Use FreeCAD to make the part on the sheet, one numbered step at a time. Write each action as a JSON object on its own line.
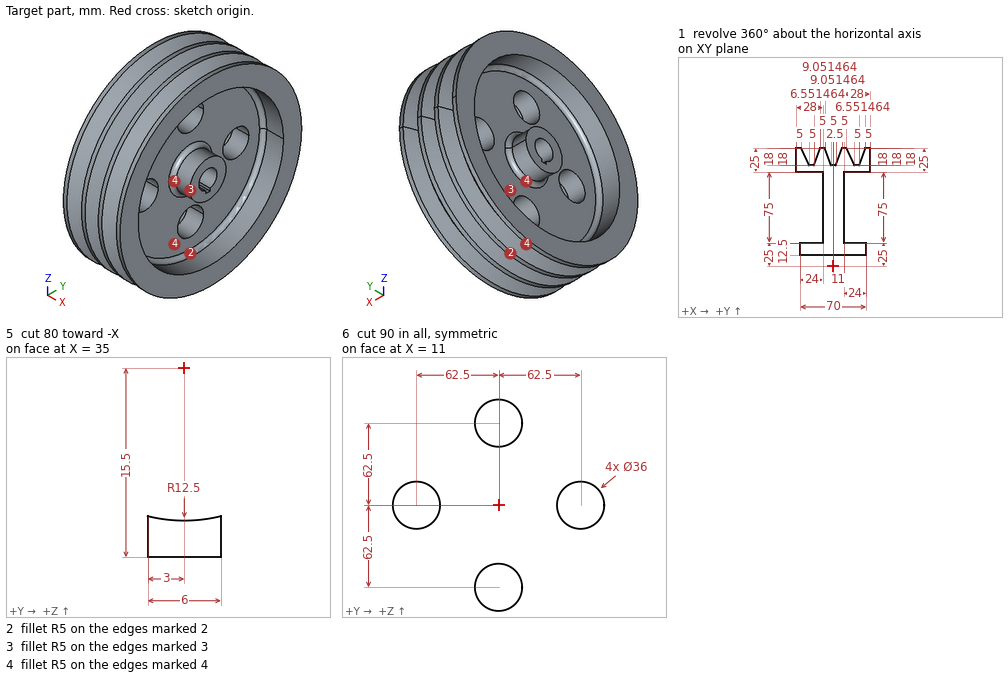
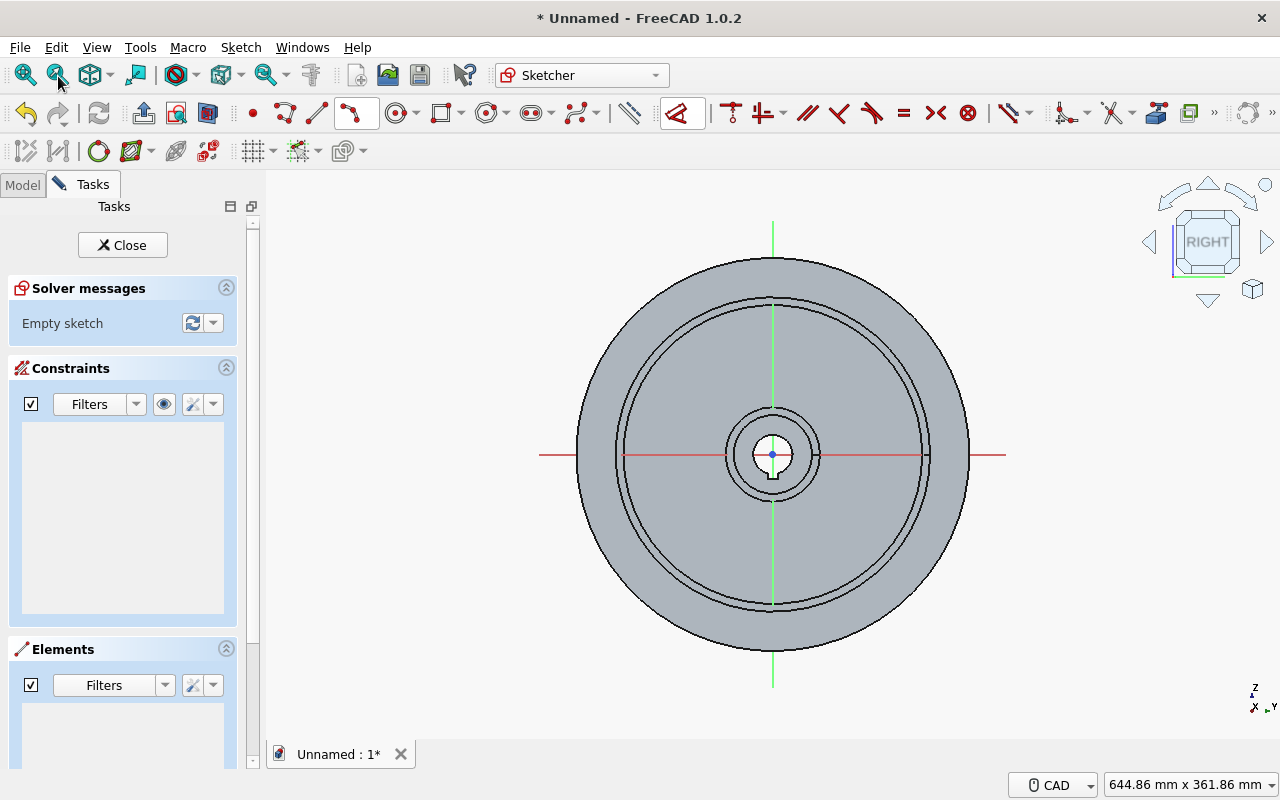
{"action": "scroll", "coordinate": [912, 454], "scroll_direction": "up", "scroll_amount": 2}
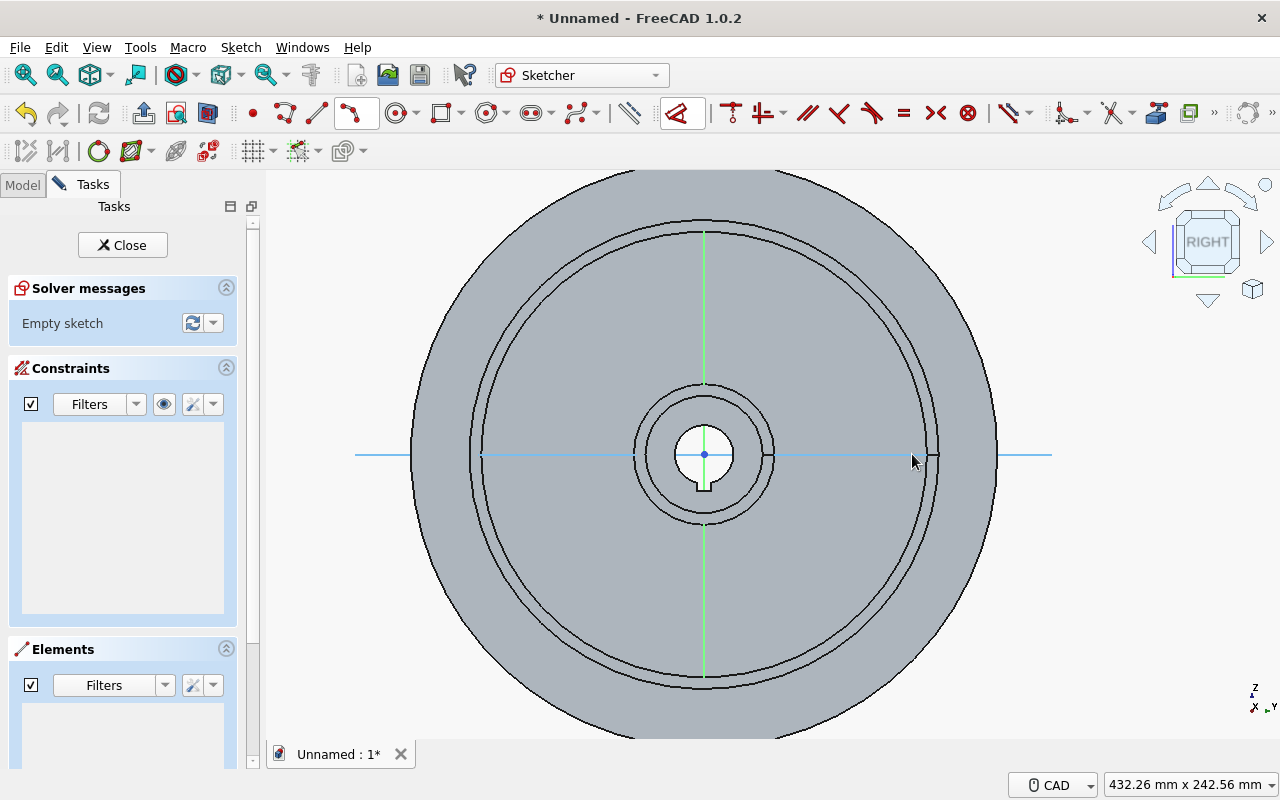
{"action": "left_click", "coordinate": [396, 114]}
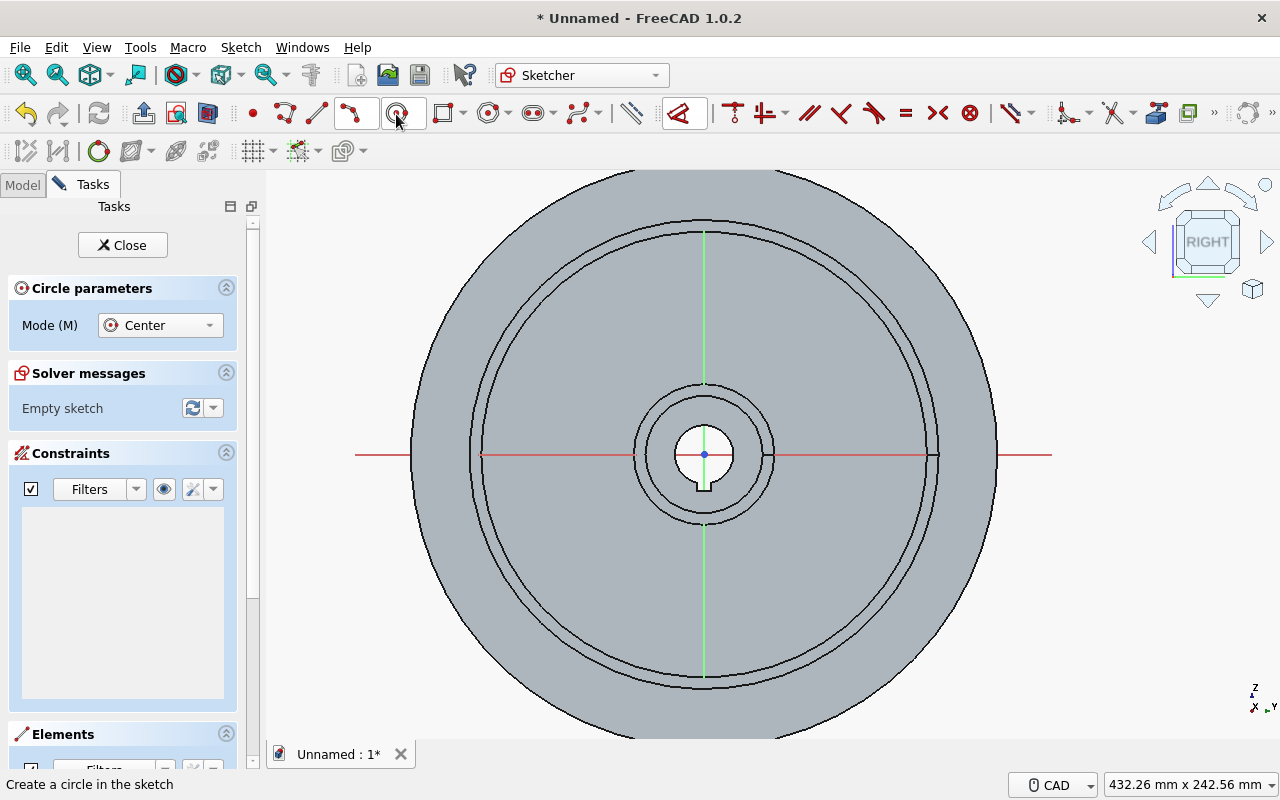
{"action": "left_click", "coordinate": [851, 454]}
{"action": "mouse_move", "coordinate": [881, 425]}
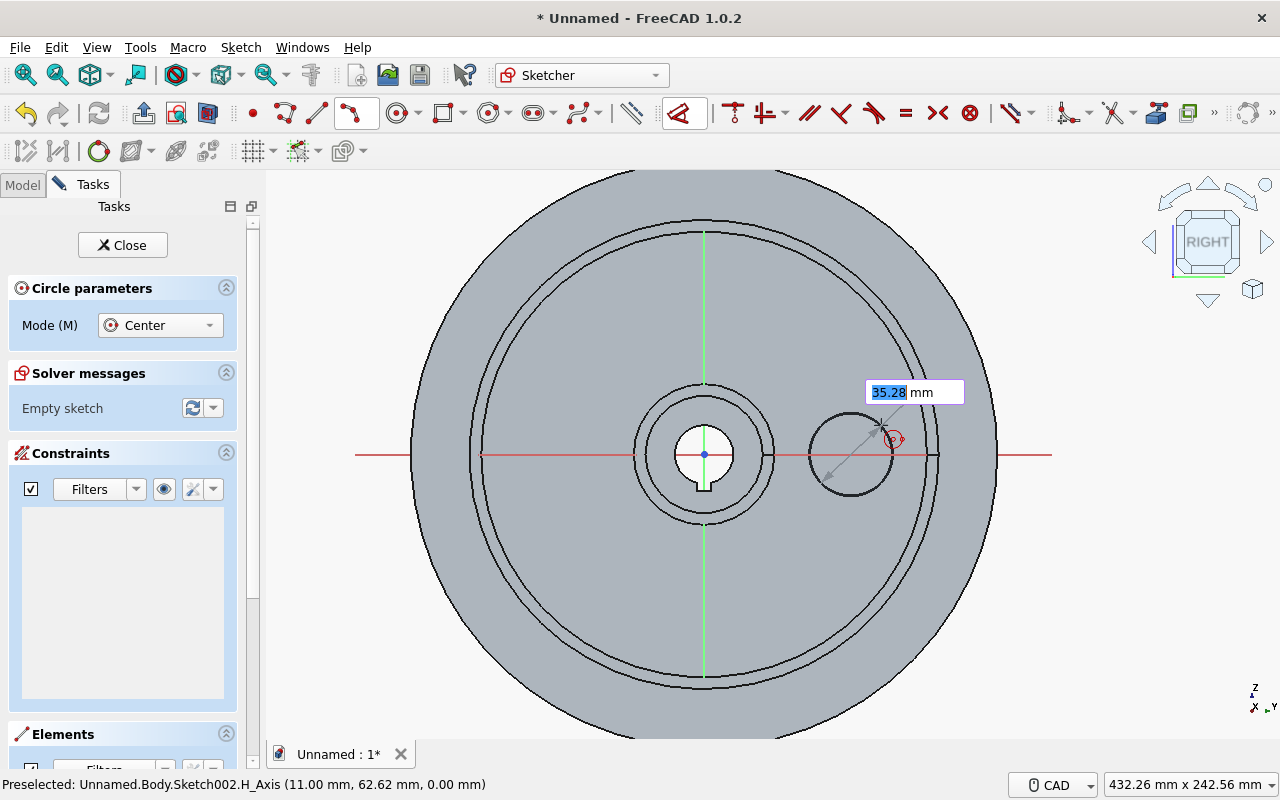
{"action": "type", "text": "36"}
{"action": "key", "text": "Return"}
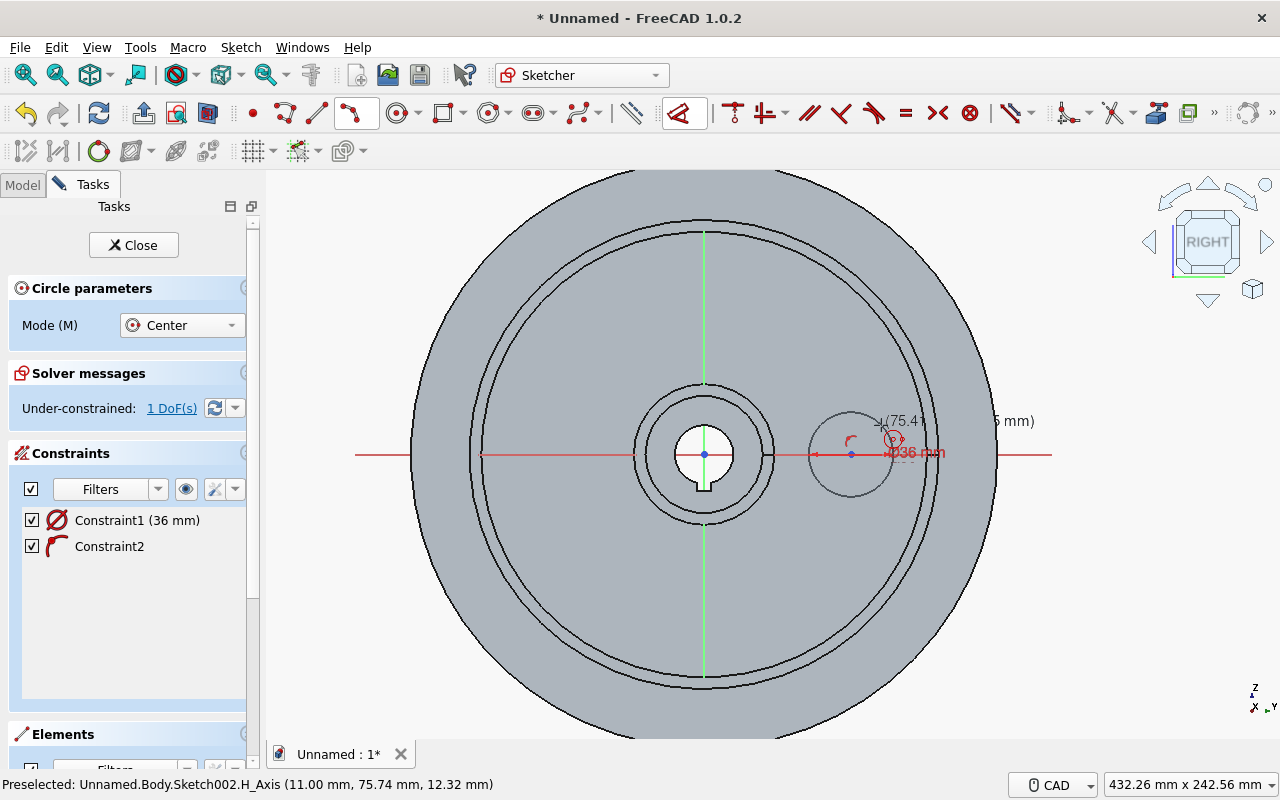
{"action": "left_click", "coordinate": [704, 601]}
{"action": "mouse_move", "coordinate": [734, 571]}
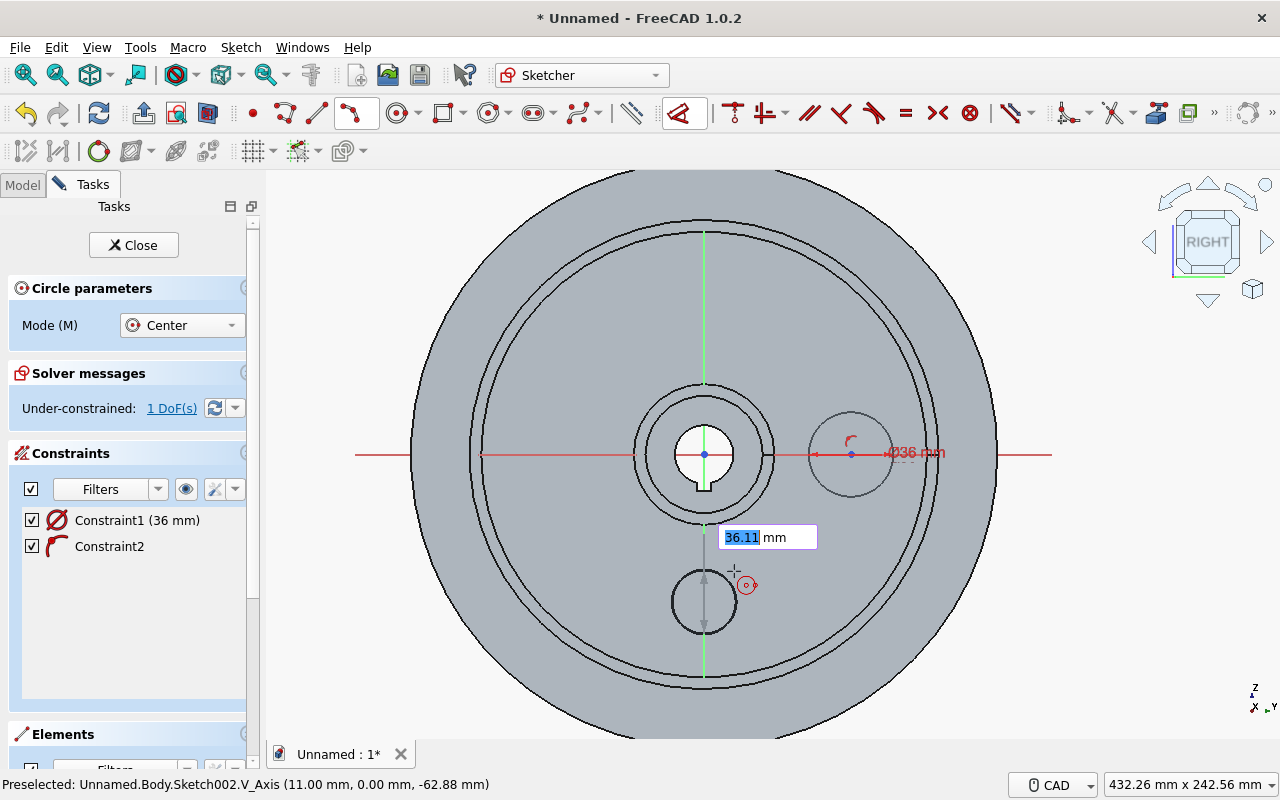
{"action": "type", "text": "36"}
{"action": "key", "text": "Return"}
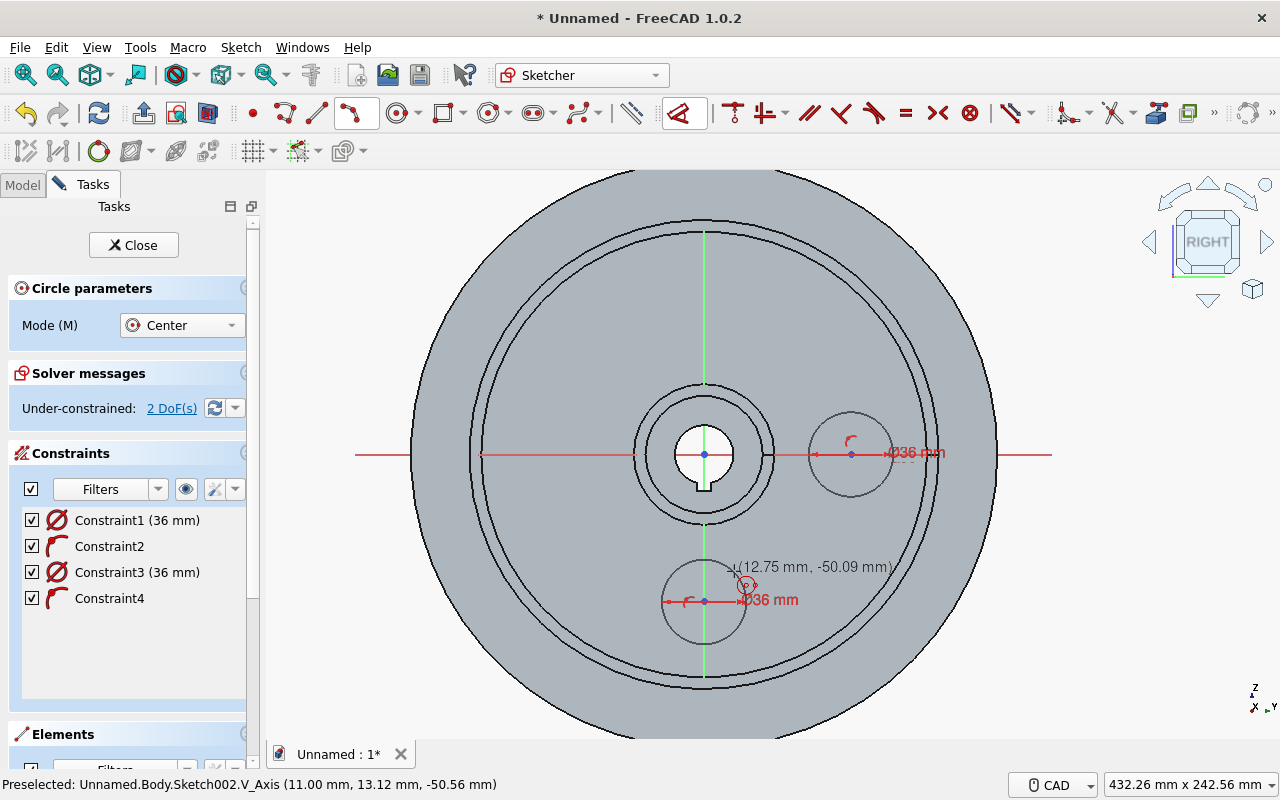
{"action": "left_click", "coordinate": [557, 454]}
{"action": "mouse_move", "coordinate": [587, 425]}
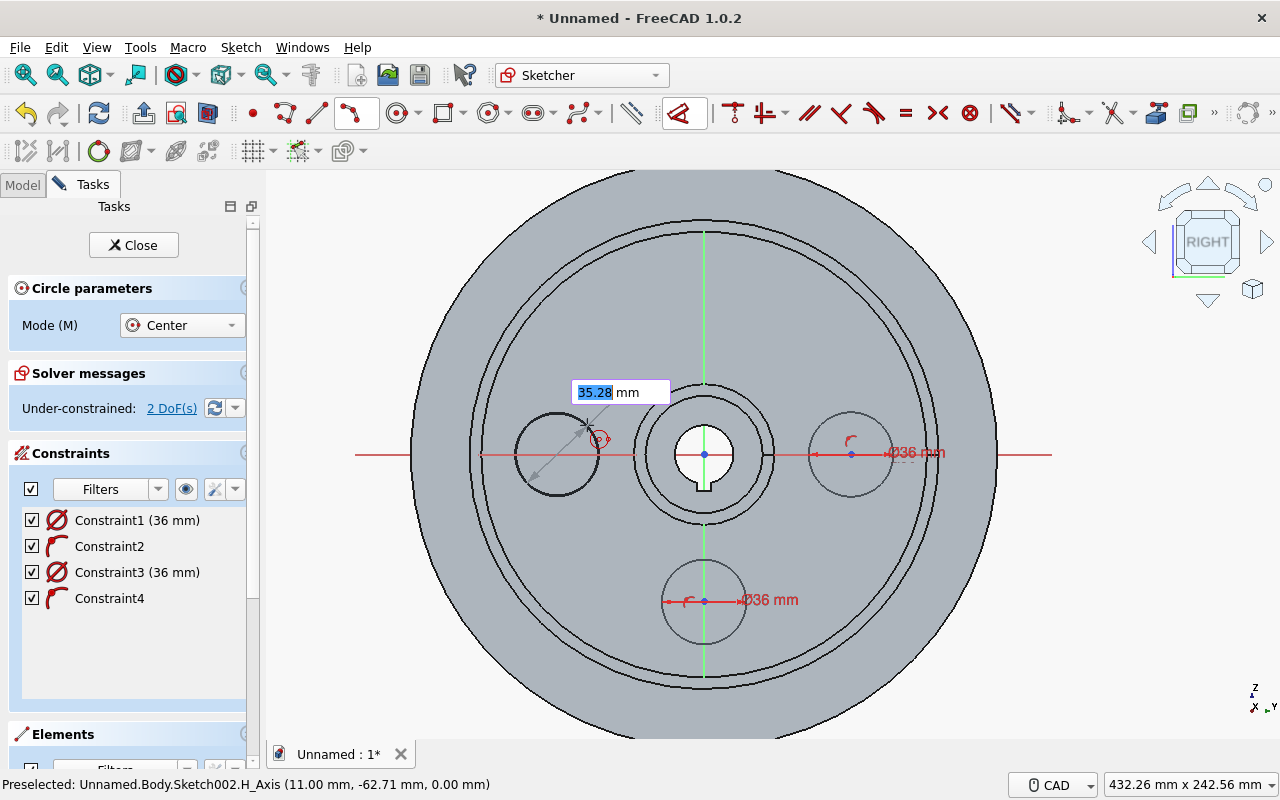
{"action": "type", "text": "36"}
{"action": "key", "text": "Return"}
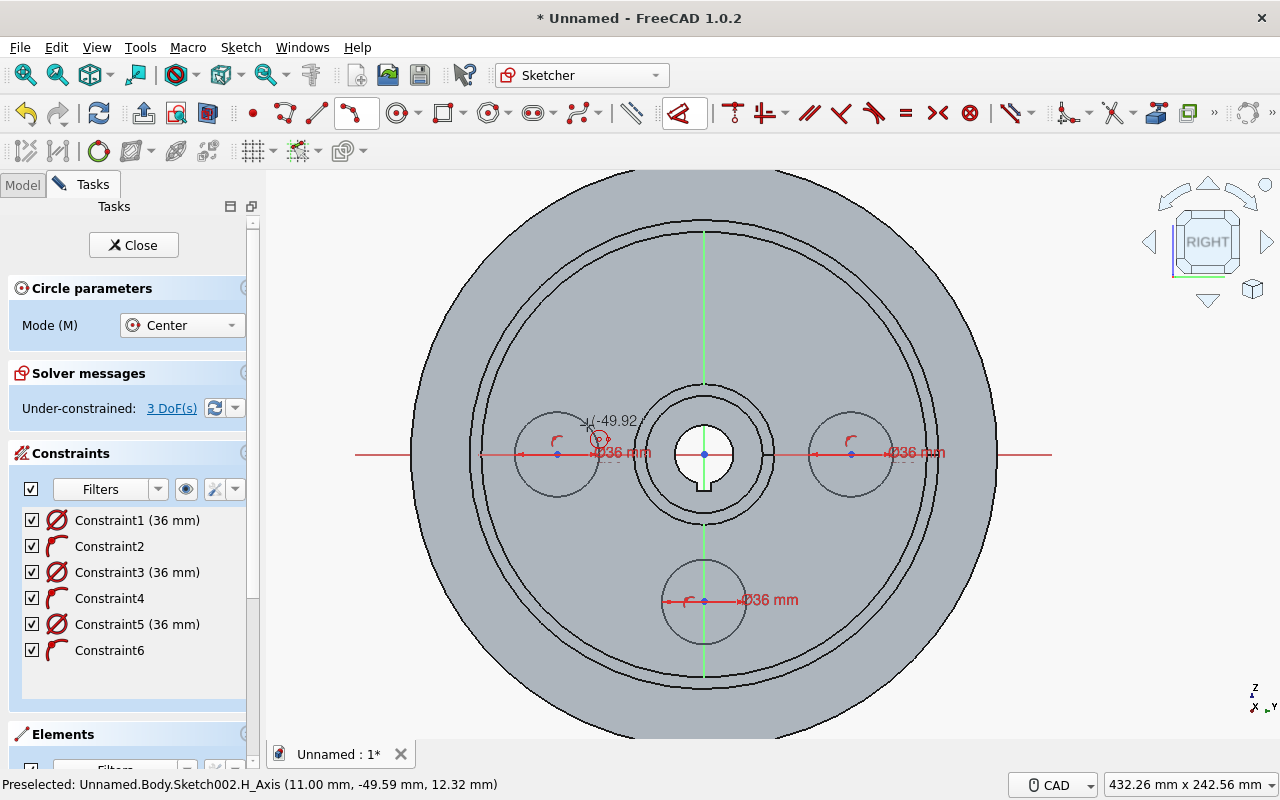
{"action": "left_click", "coordinate": [704, 308]}
{"action": "mouse_move", "coordinate": [734, 278]}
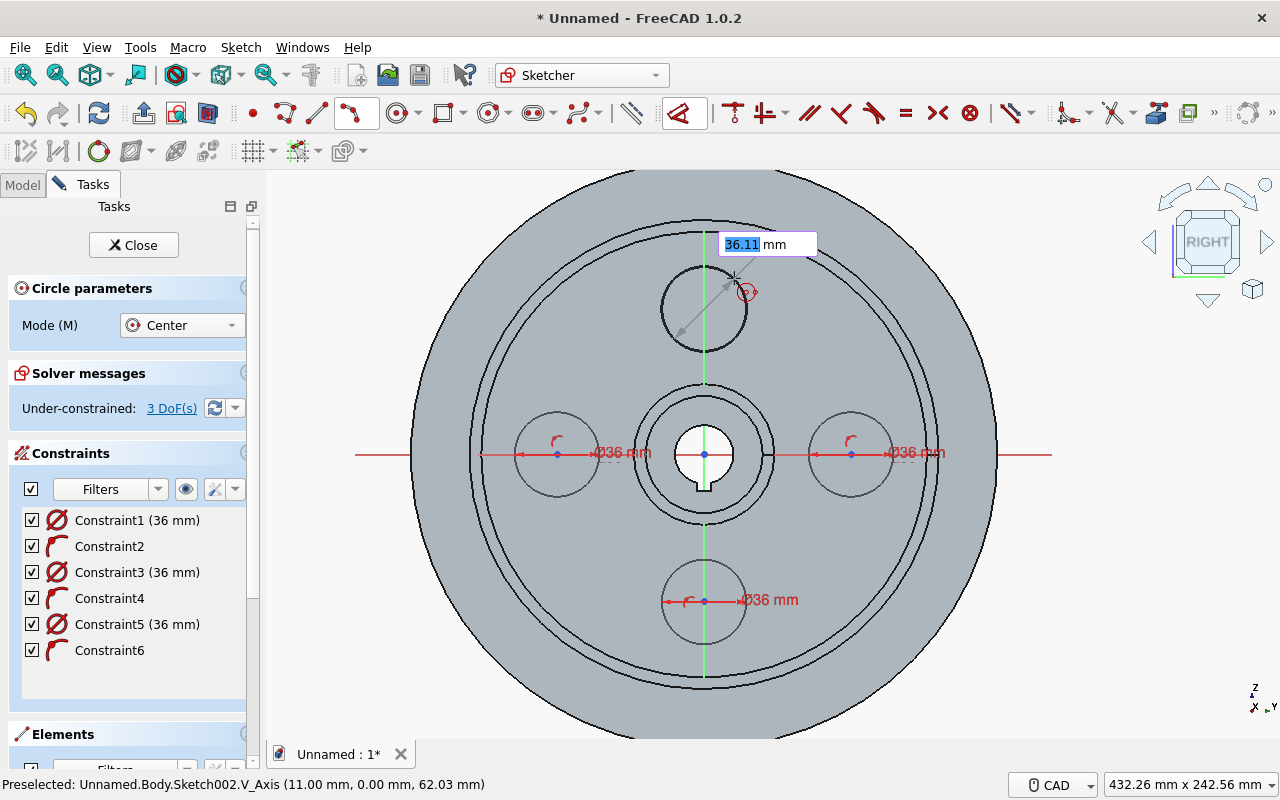
{"action": "type", "text": "36"}
{"action": "key", "text": "Return"}
{"action": "key", "text": "Escape"}